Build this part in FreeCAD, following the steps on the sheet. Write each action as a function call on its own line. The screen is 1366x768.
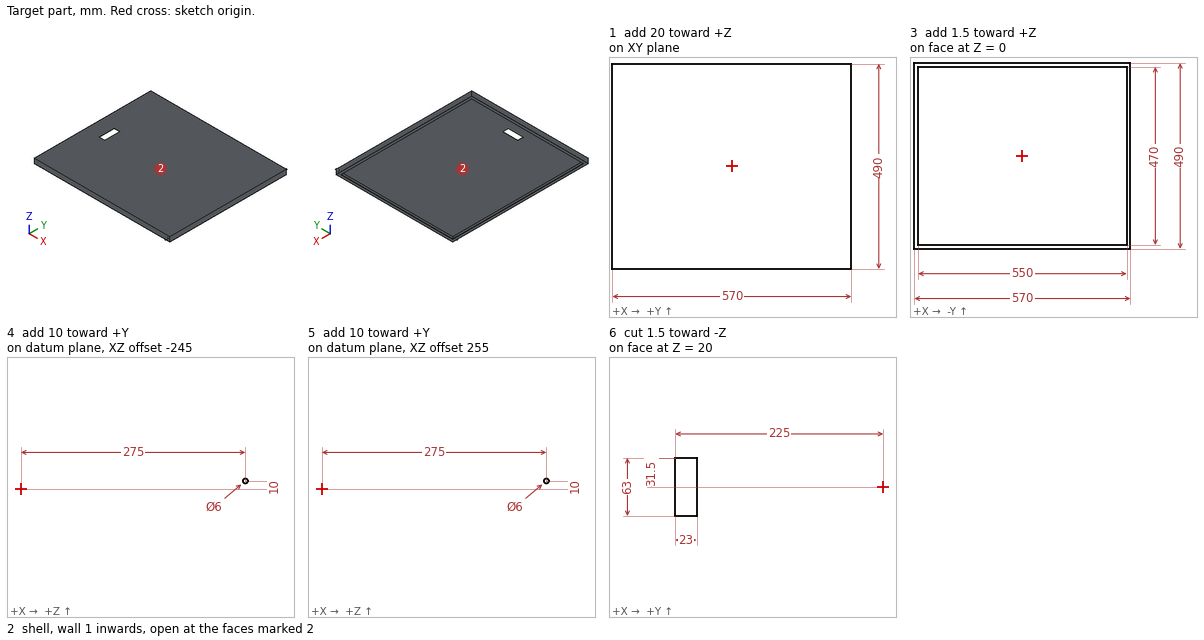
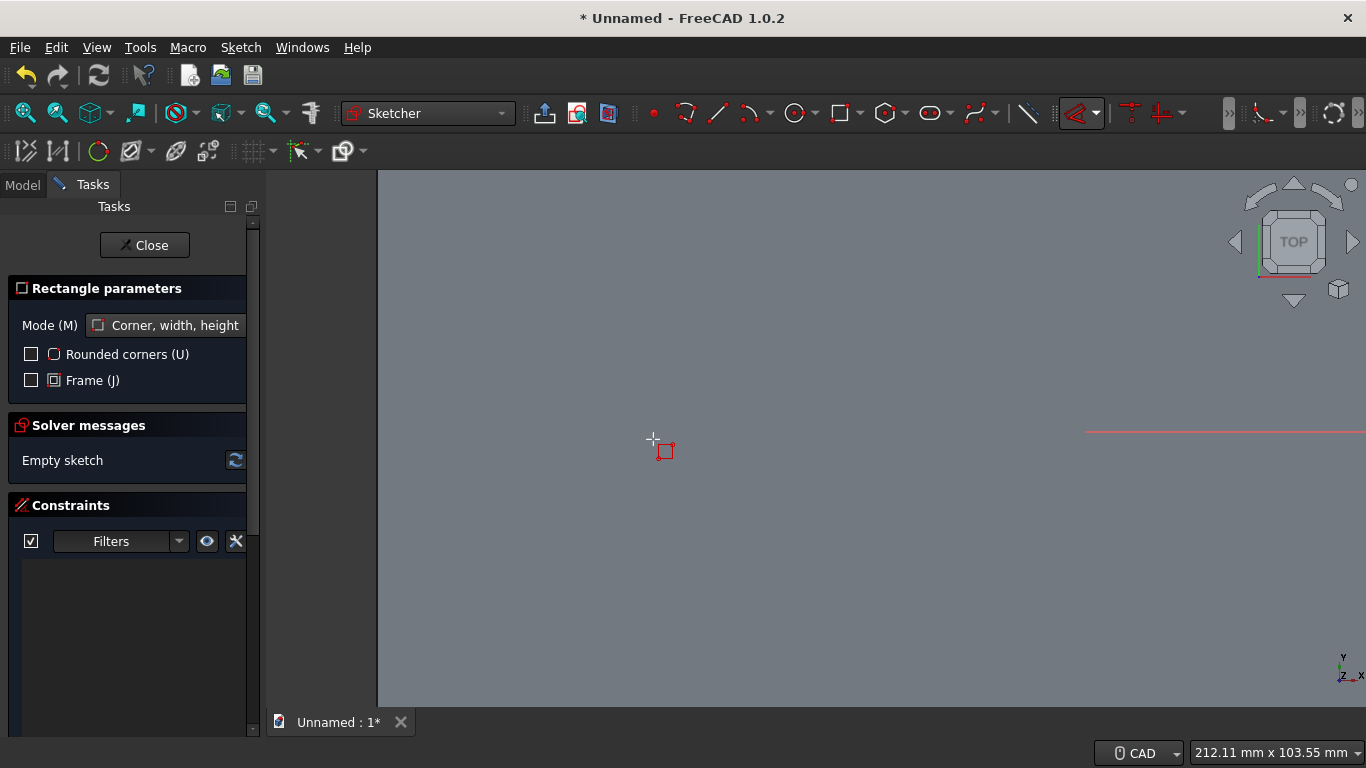
click(688, 269)
click(808, 595)
key(Escape)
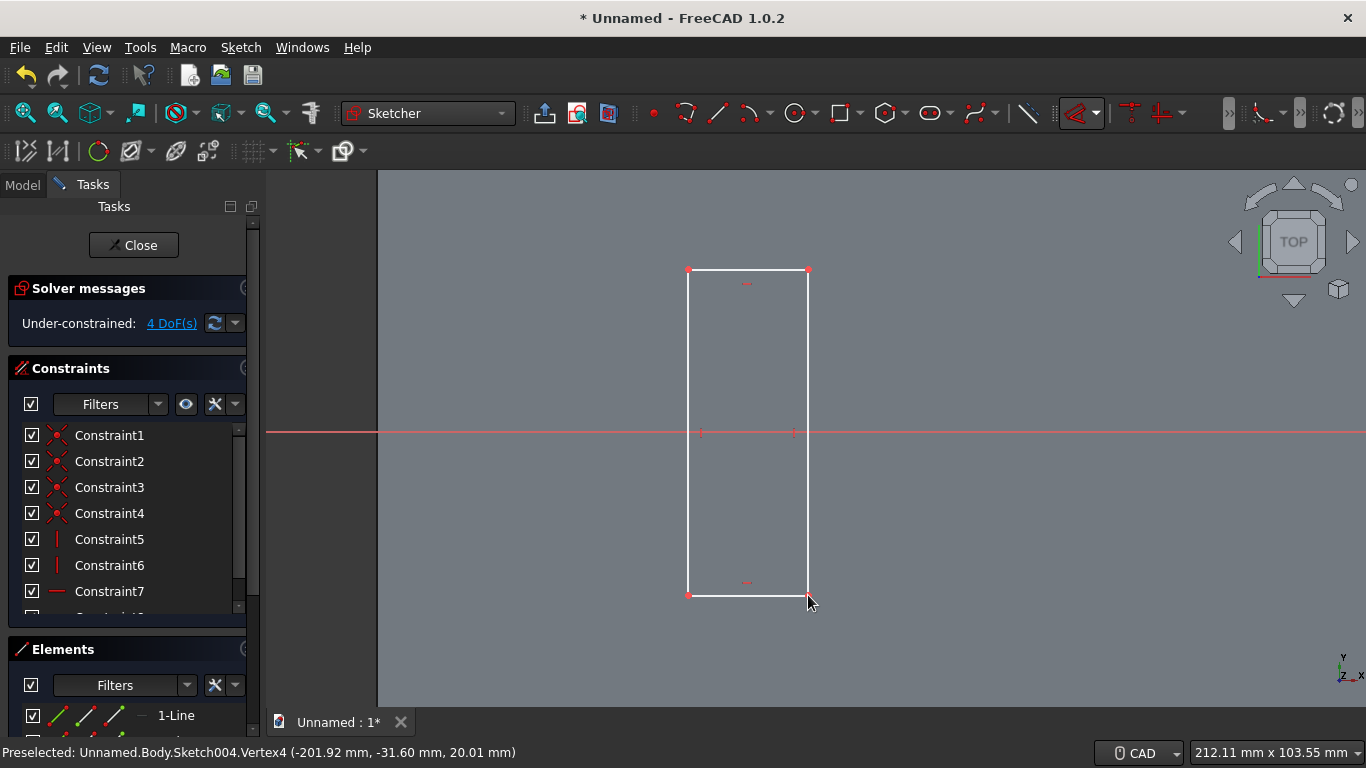
click(688, 368)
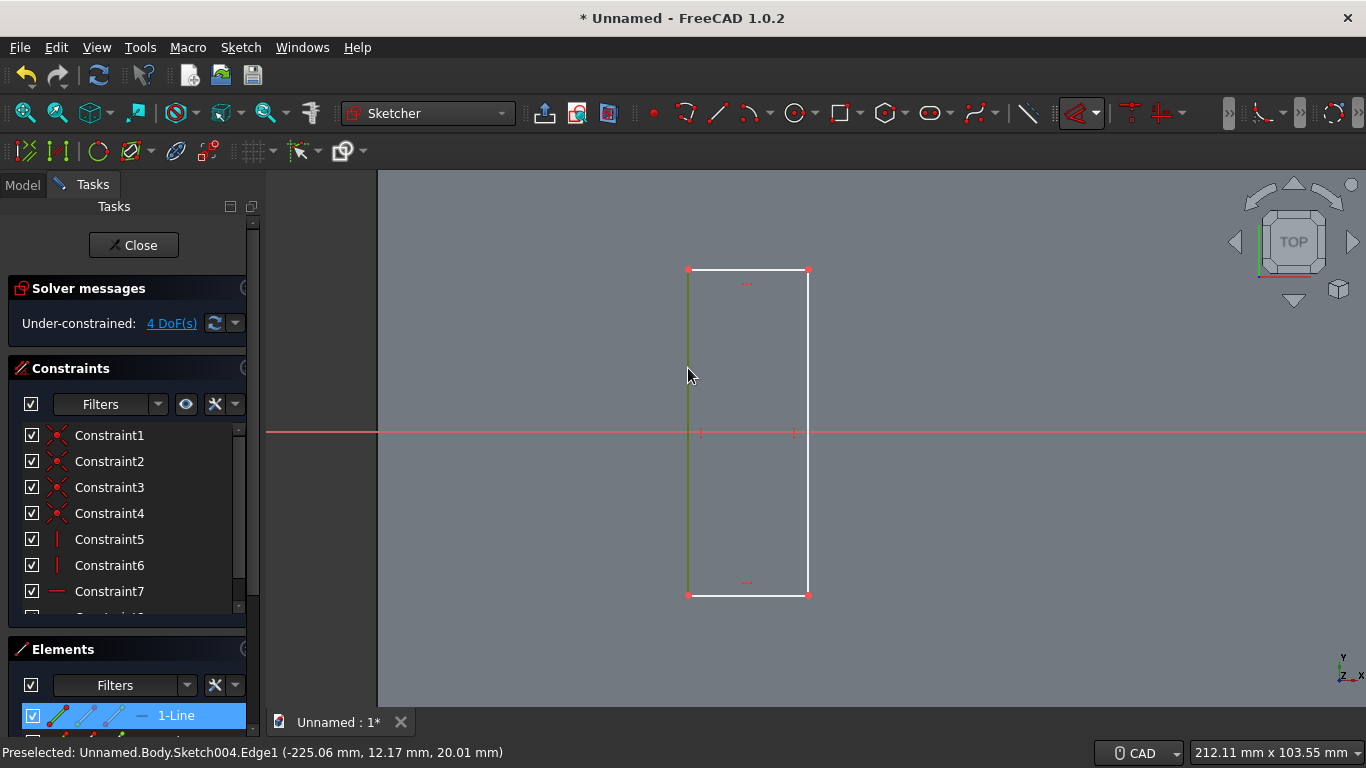
key(i)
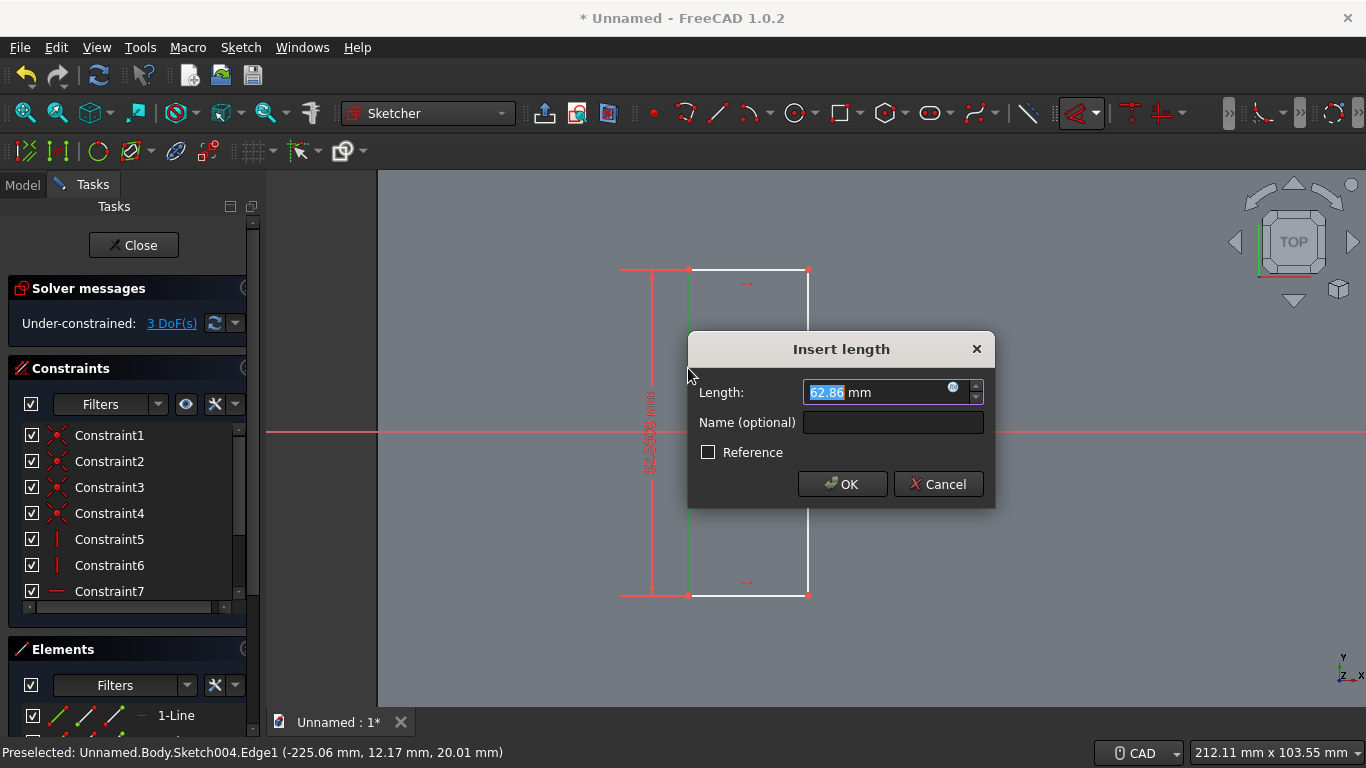
text(63)
key(Return)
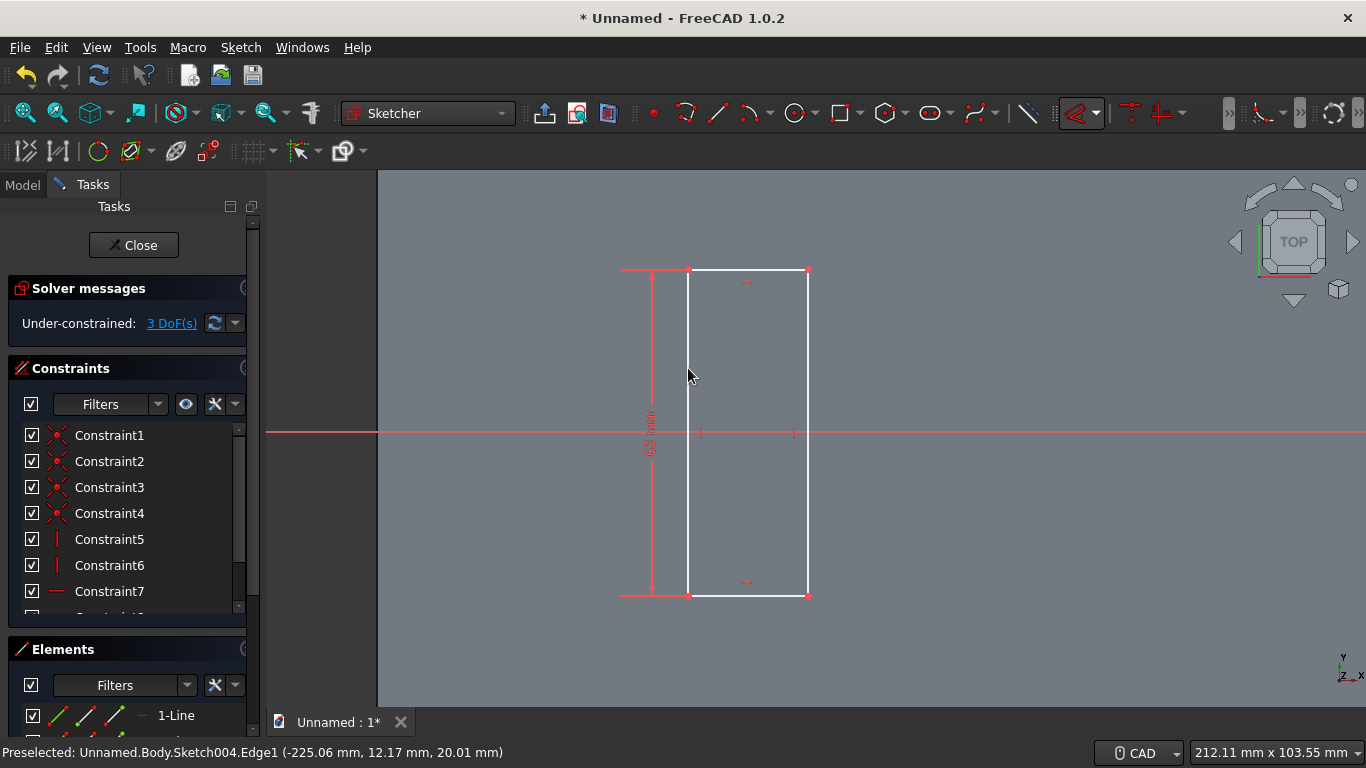
click(724, 596)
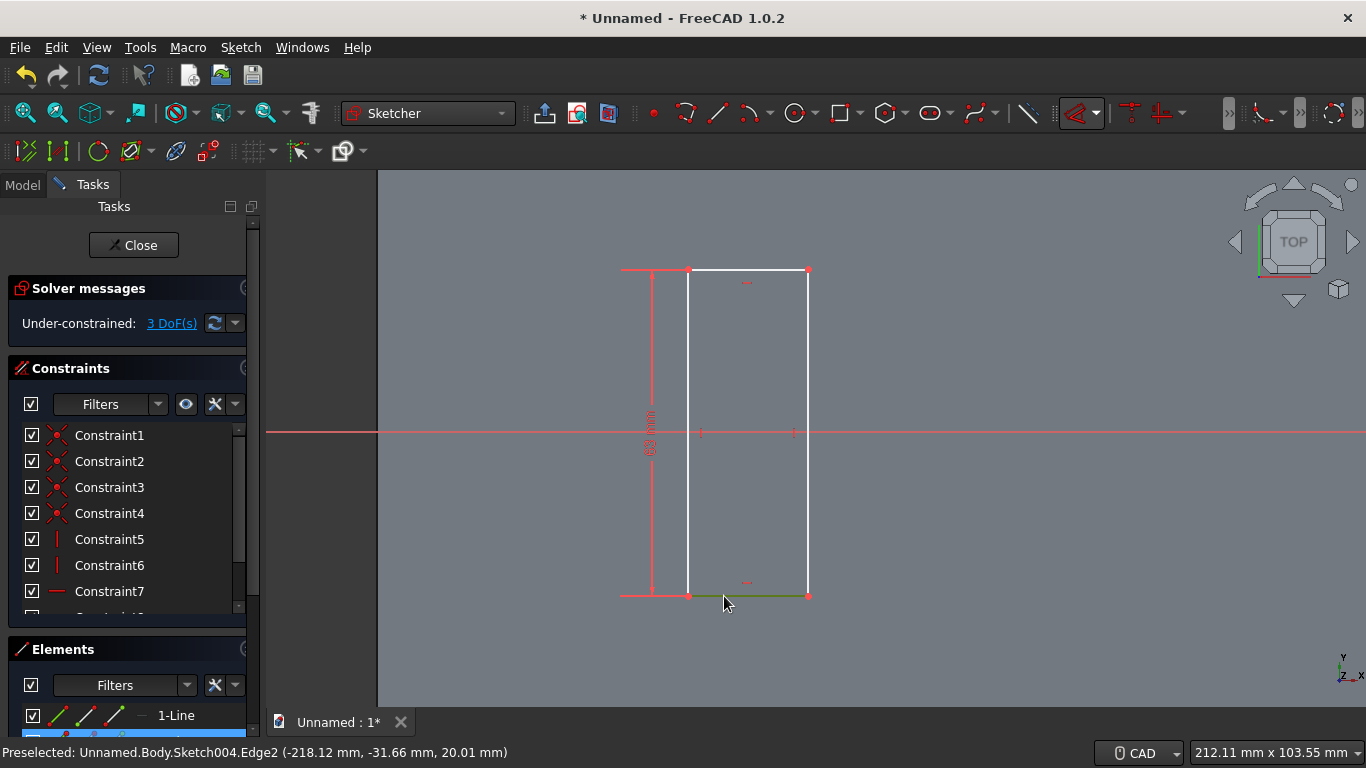
key(l)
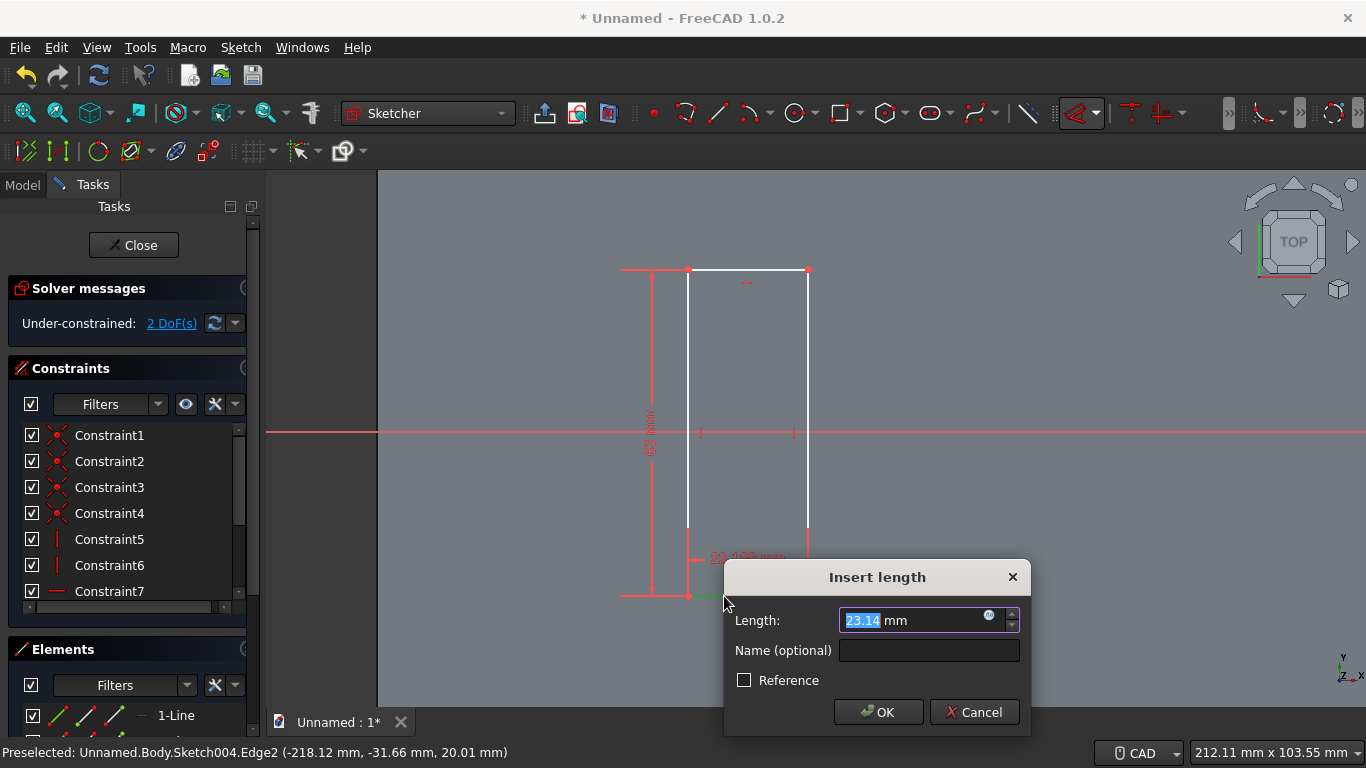
text(23)
key(Return)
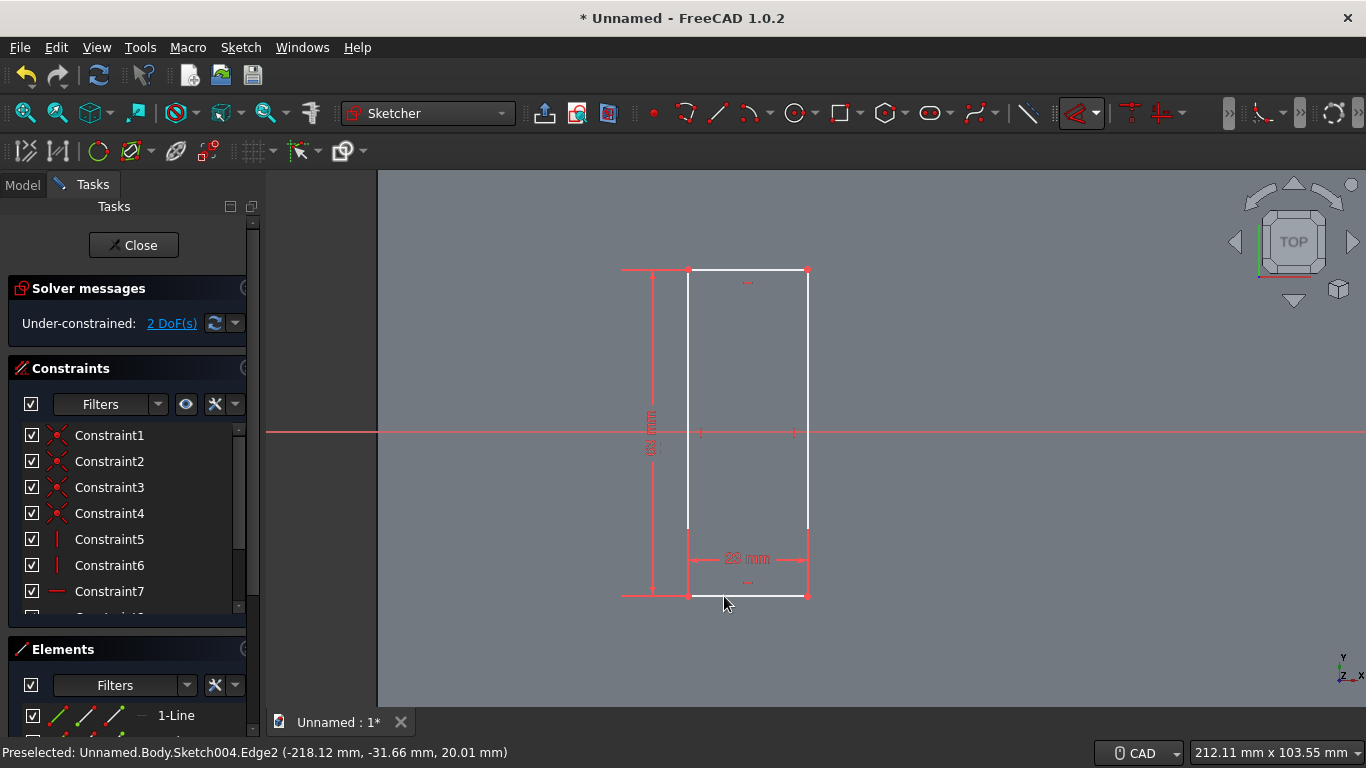
click(688, 270)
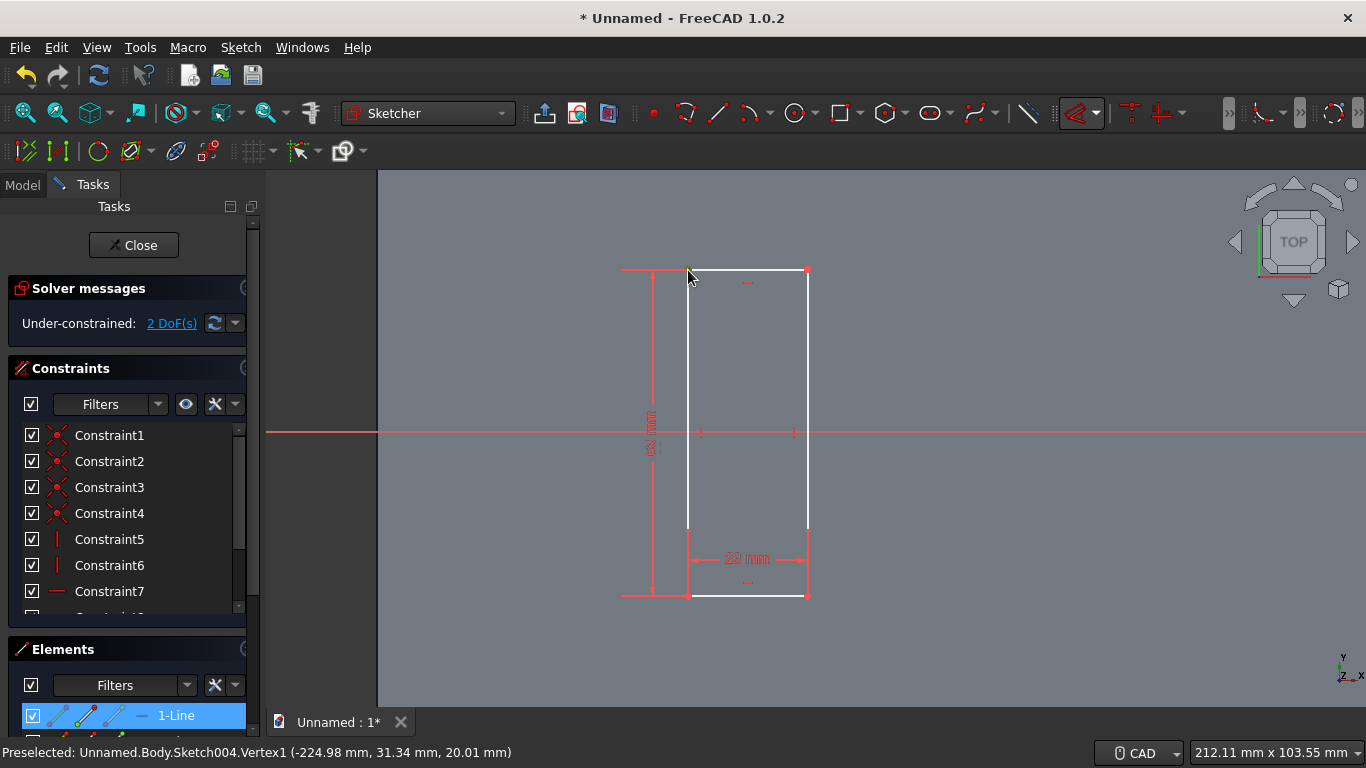
key(l)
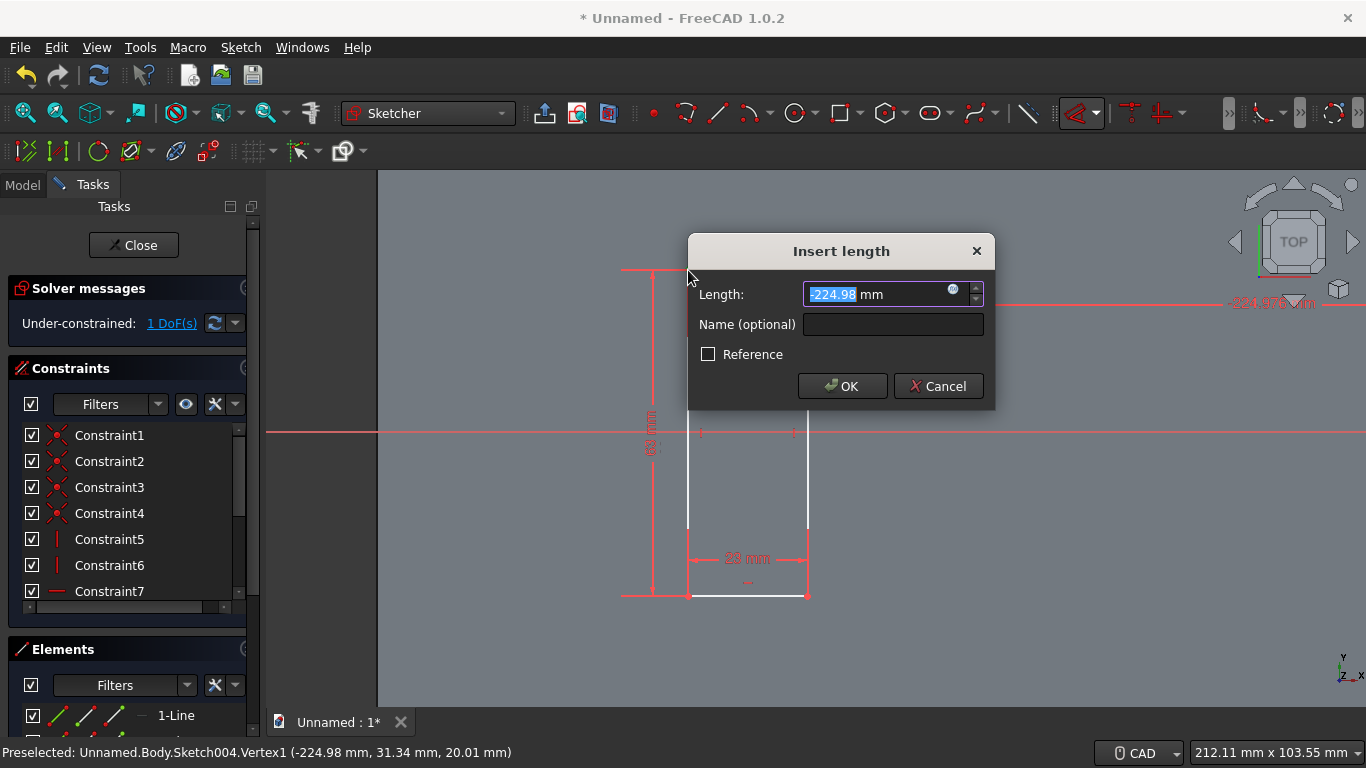
text(-225)
key(Return)